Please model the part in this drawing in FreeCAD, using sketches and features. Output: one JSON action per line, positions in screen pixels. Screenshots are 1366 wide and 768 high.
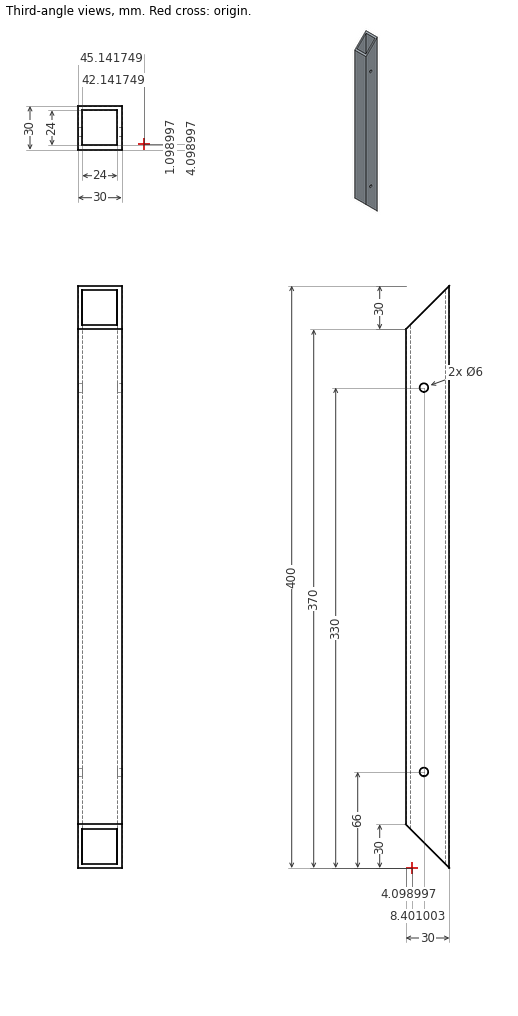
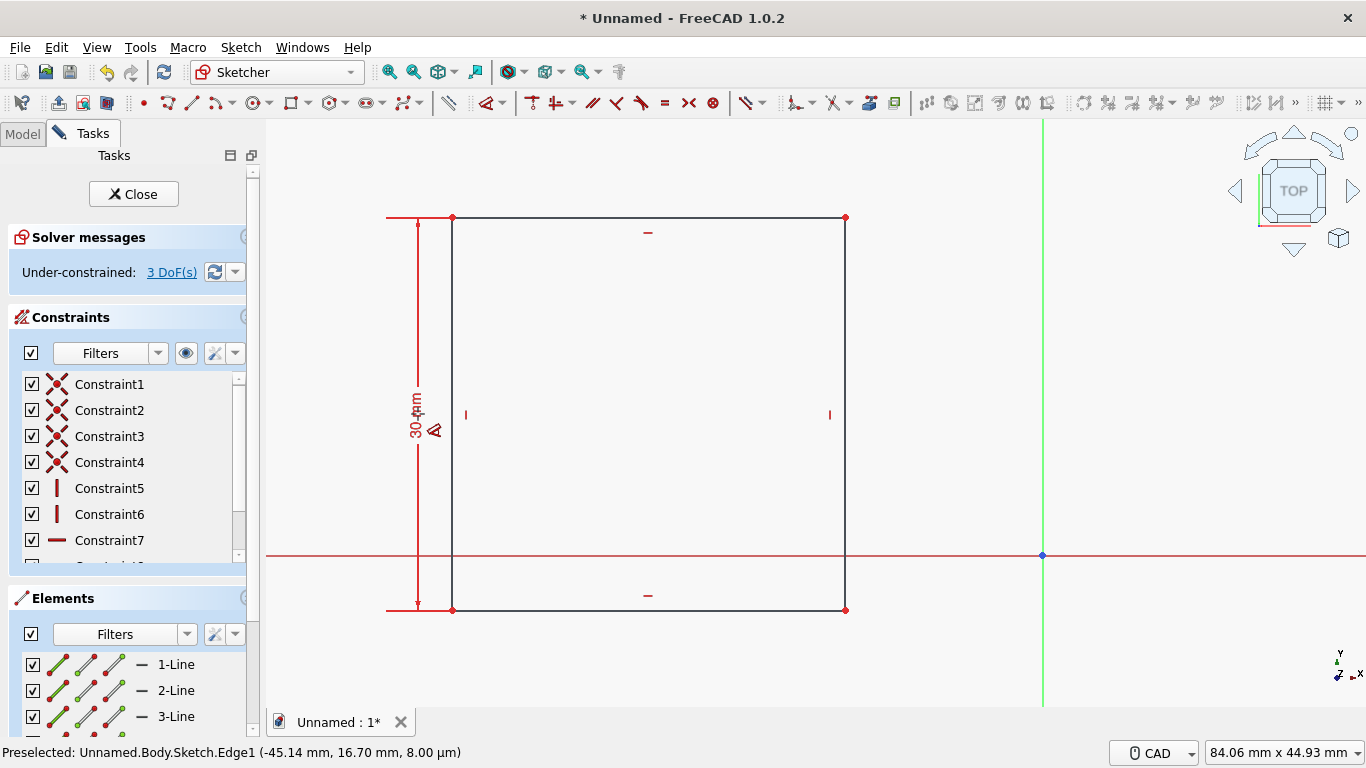
{"action": "left_click", "coordinate": [570, 611]}
{"action": "left_click", "coordinate": [649, 645]}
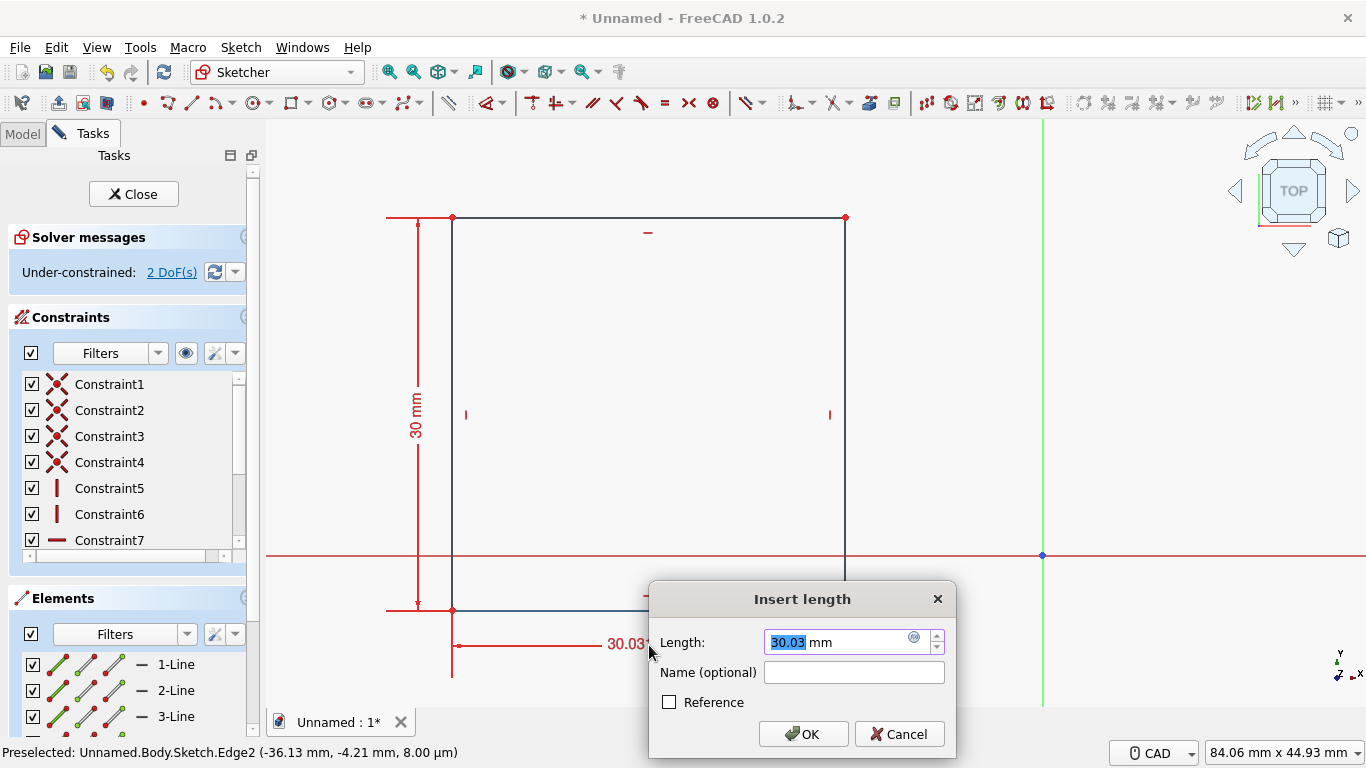
{"action": "type", "text": "30"}
{"action": "key", "text": "Return"}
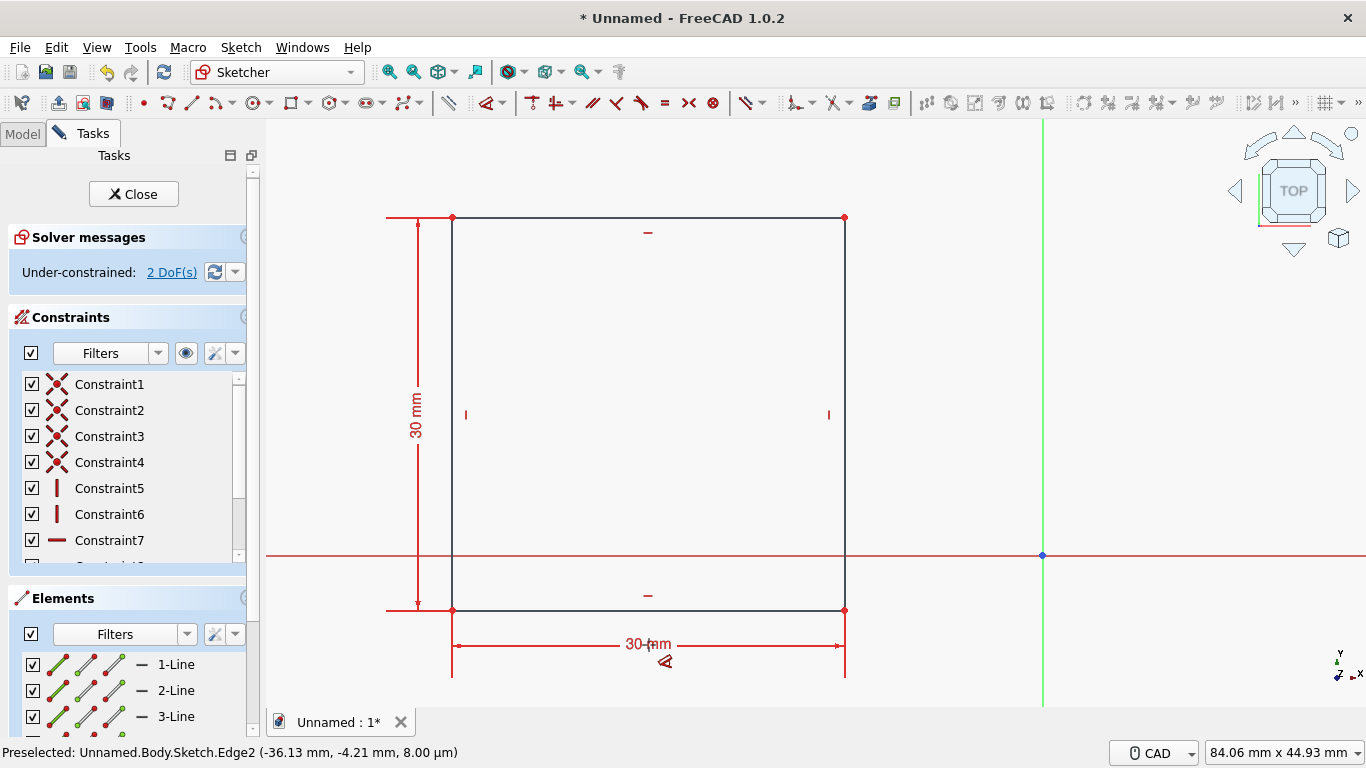
{"action": "left_click", "coordinate": [452, 611]}
{"action": "left_click", "coordinate": [418, 583]}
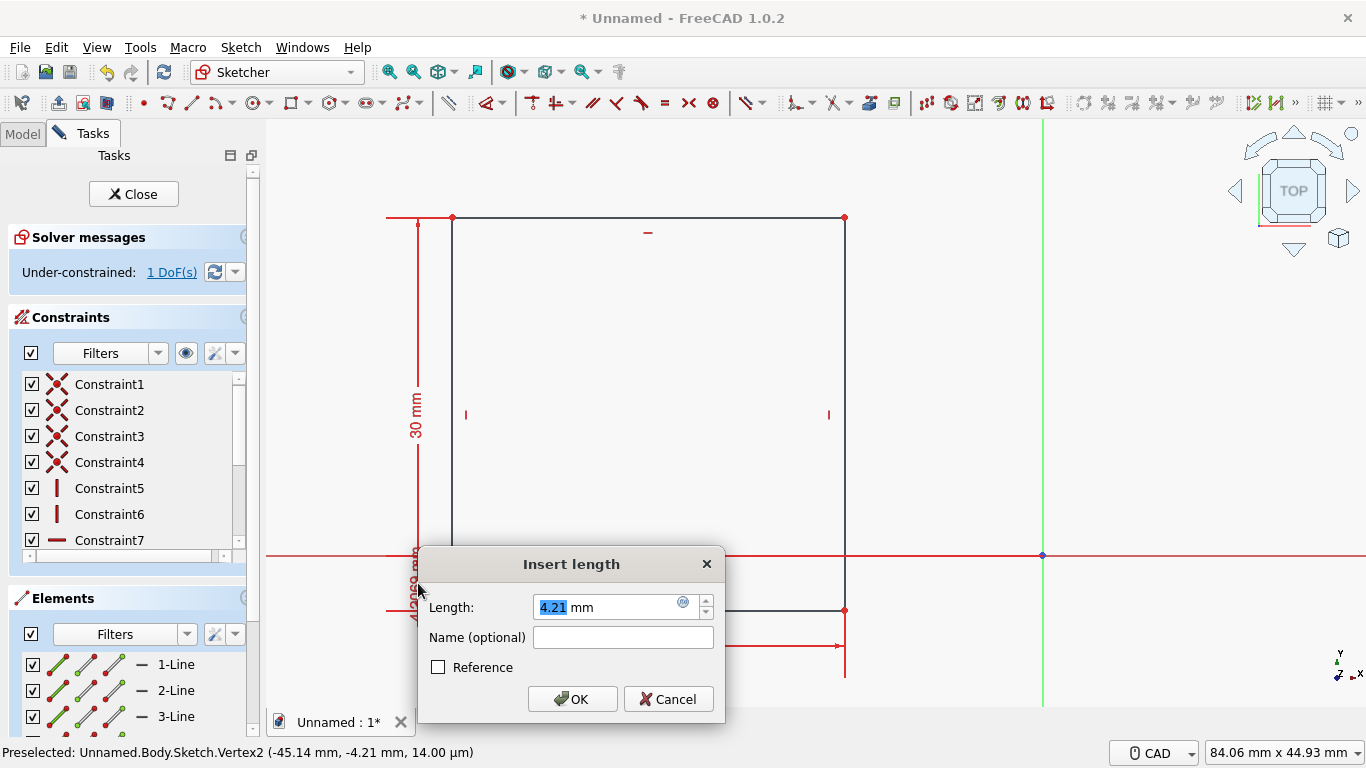
{"action": "type", "text": "4.098997"}
{"action": "key", "text": "Return"}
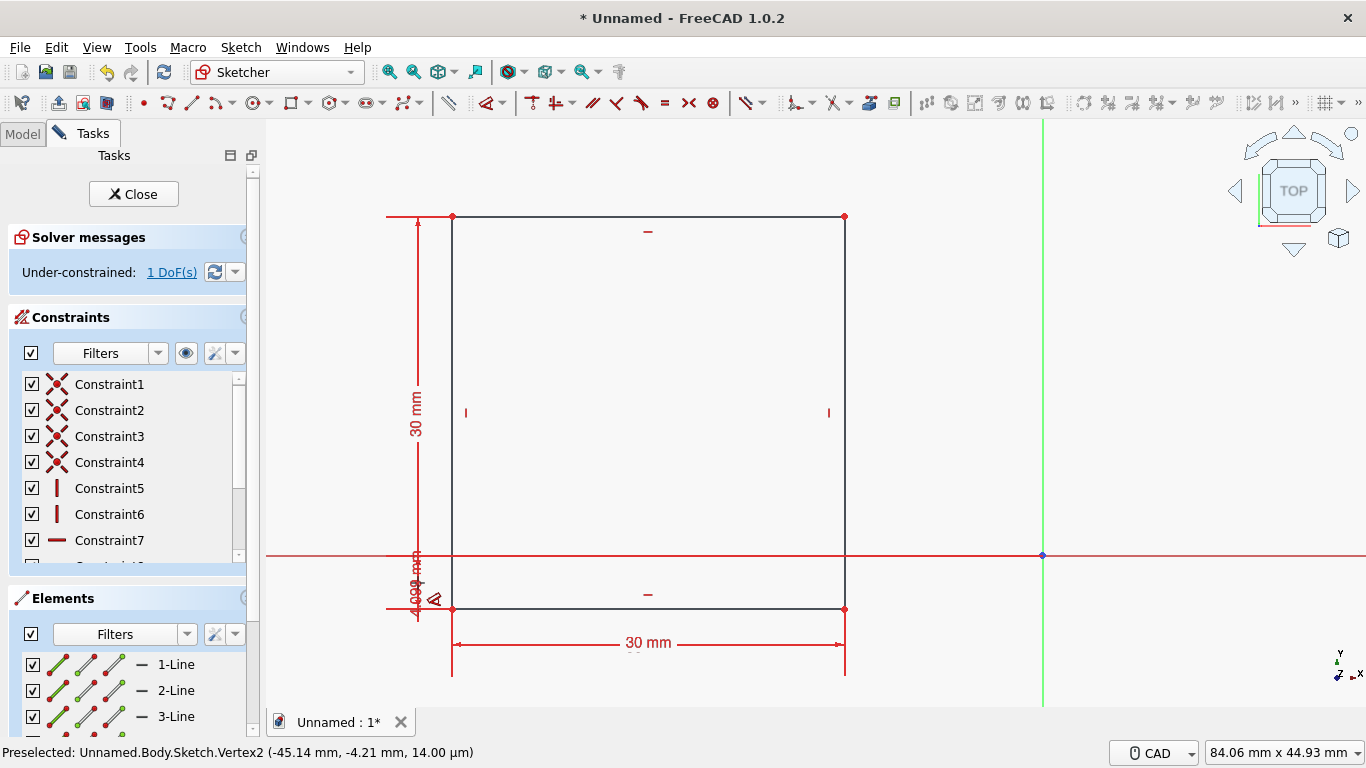
{"action": "left_click", "coordinate": [452, 217]}
{"action": "left_click", "coordinate": [747, 183]}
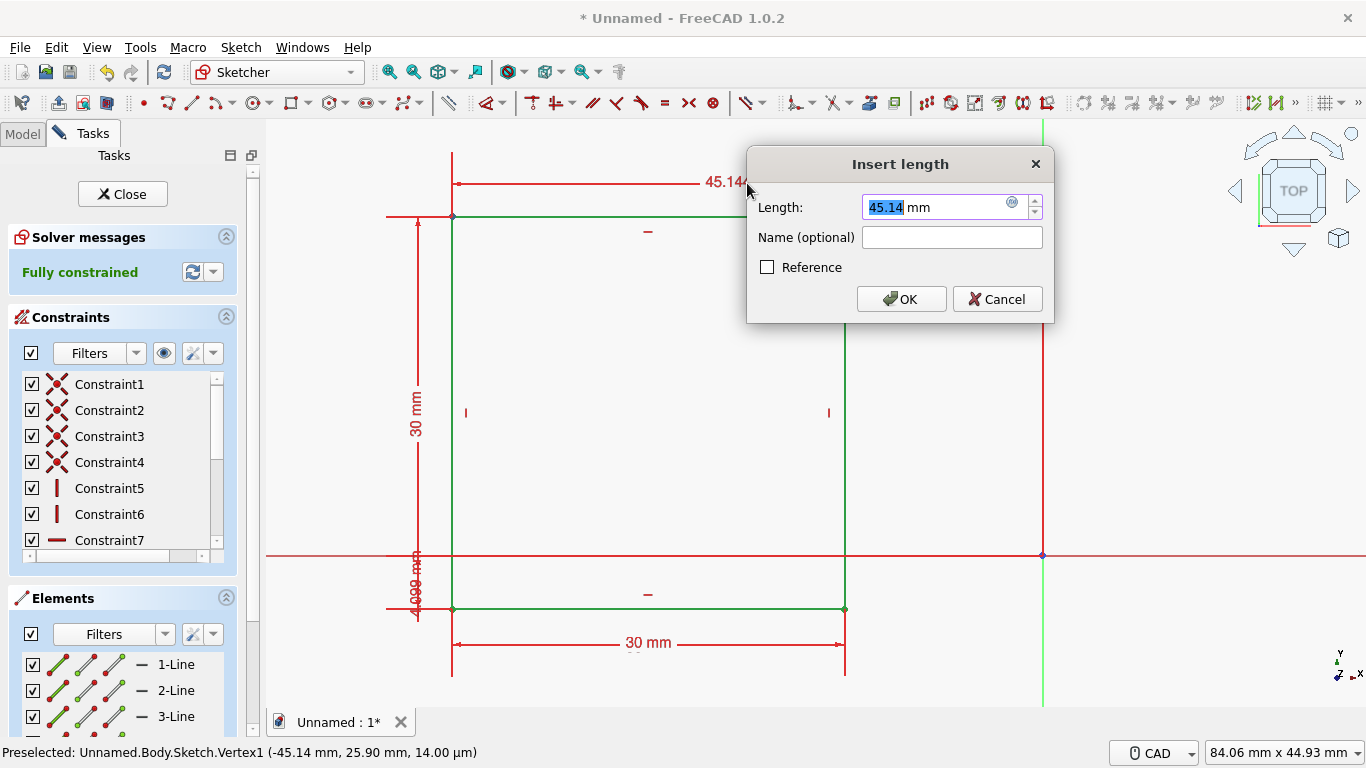
{"action": "type", "text": "45.141749"}
{"action": "key", "text": "Return"}
{"action": "key", "text": "Escape"}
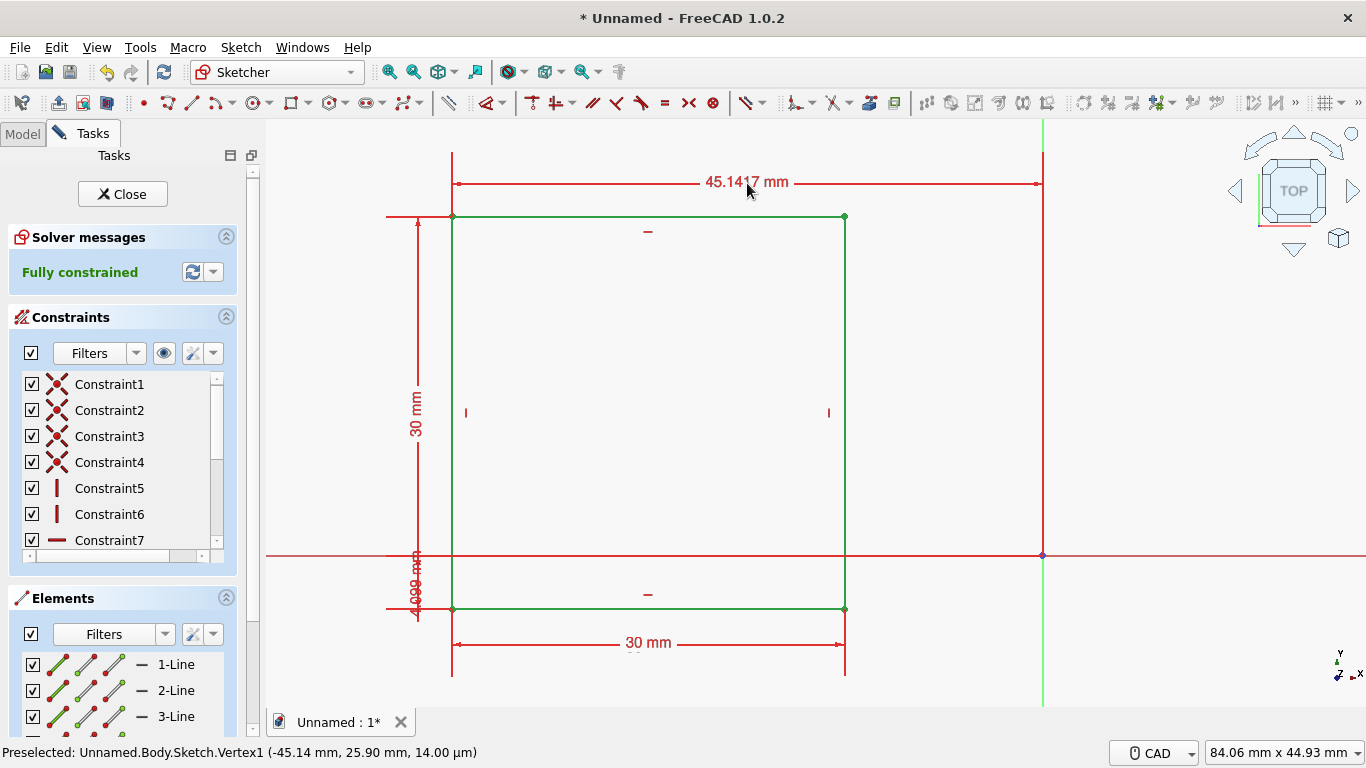
{"action": "left_click", "coordinate": [123, 194]}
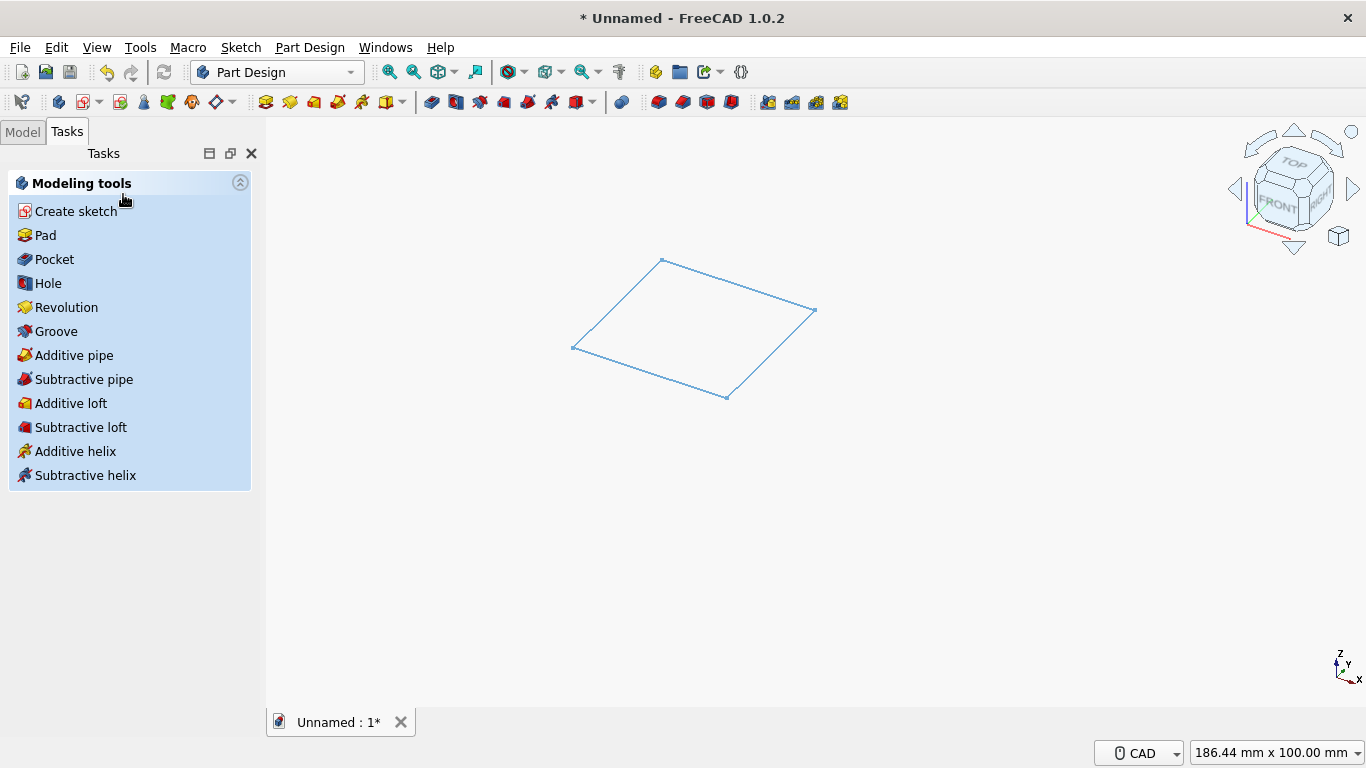
{"action": "left_click", "coordinate": [266, 102]}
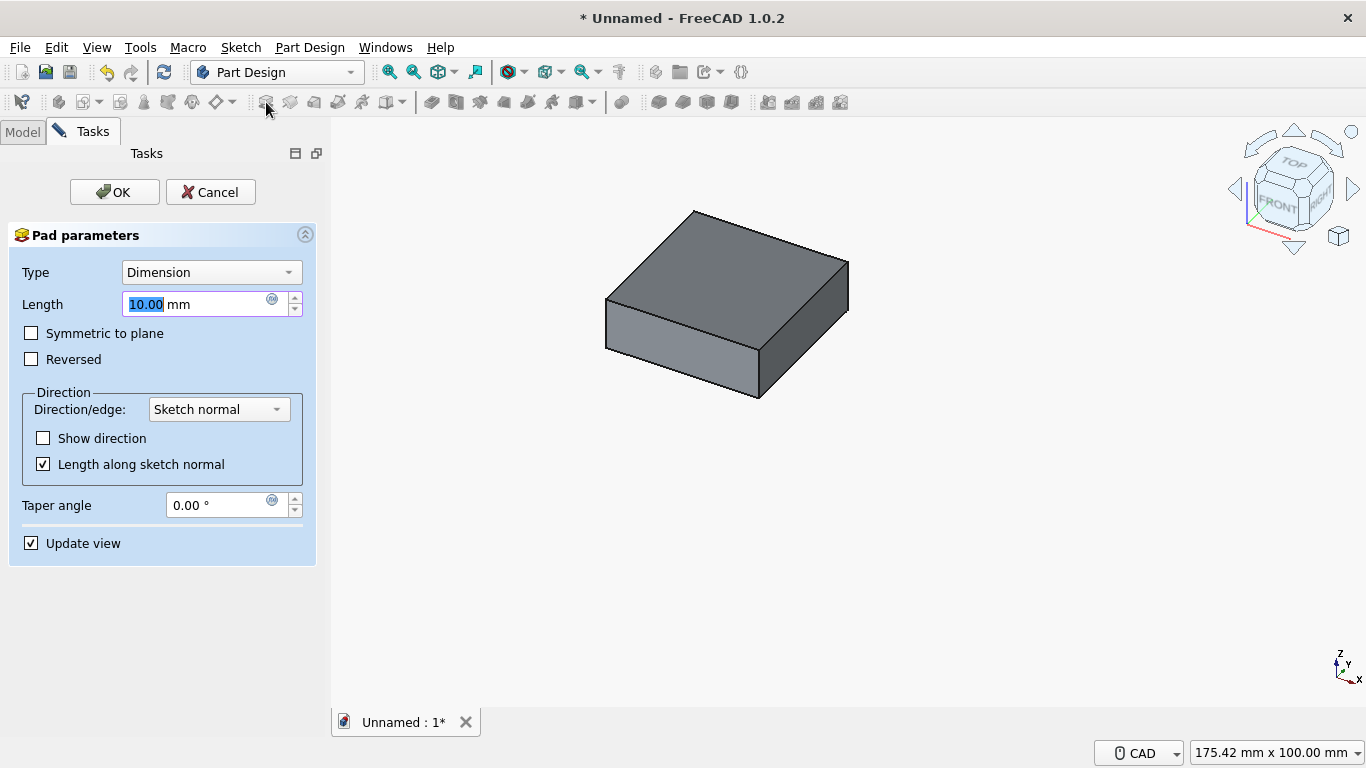
{"action": "type", "text": "400"}
{"action": "key", "text": "Tab"}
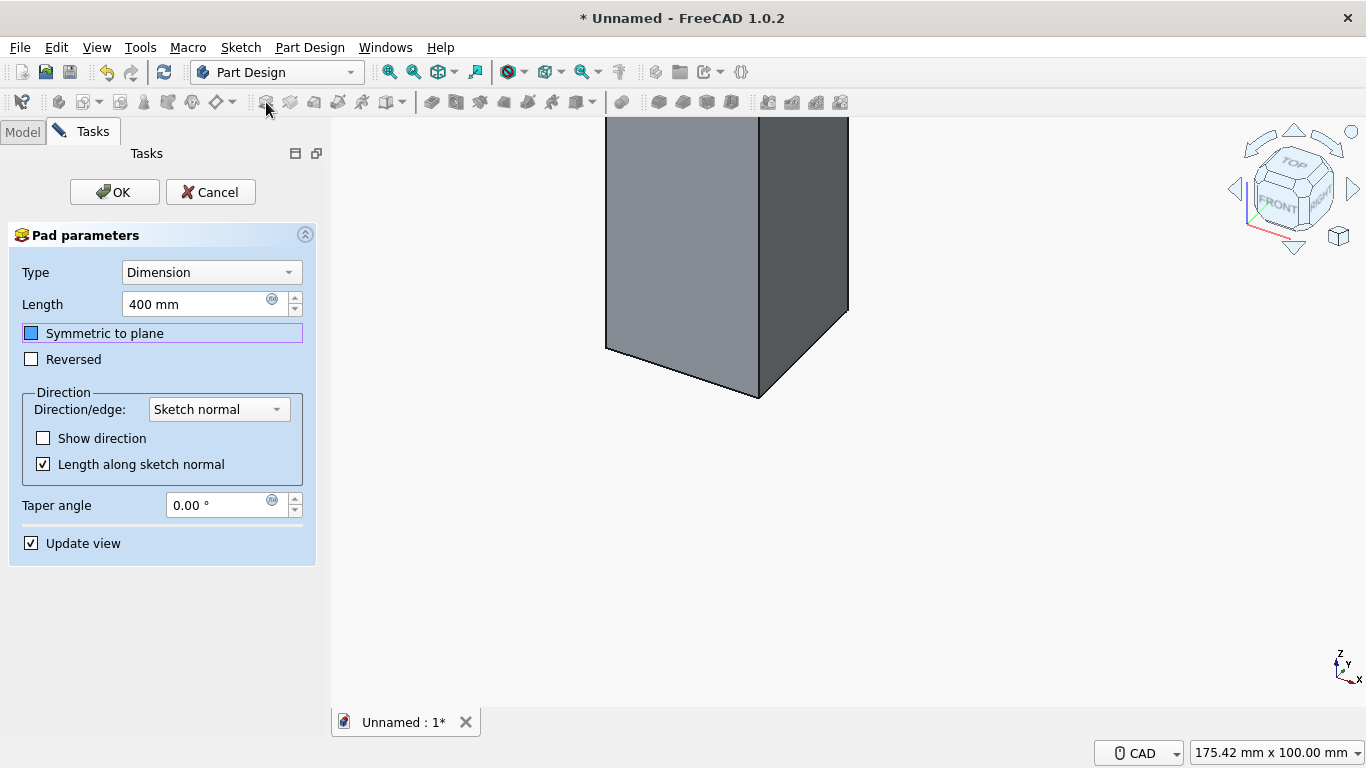
{"action": "left_click", "coordinate": [115, 192]}